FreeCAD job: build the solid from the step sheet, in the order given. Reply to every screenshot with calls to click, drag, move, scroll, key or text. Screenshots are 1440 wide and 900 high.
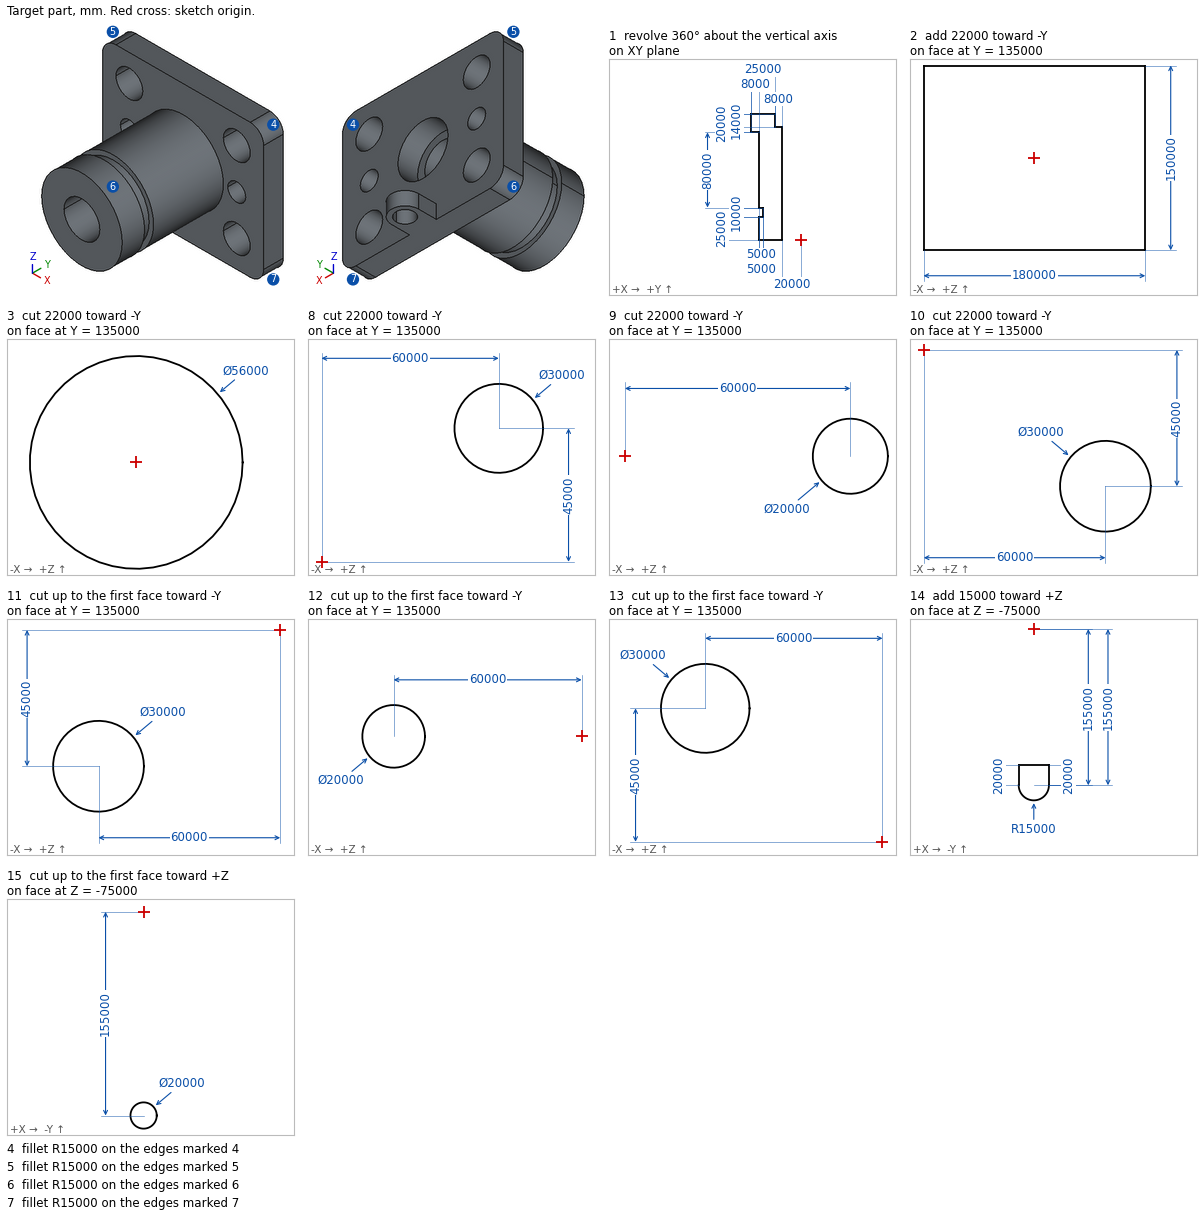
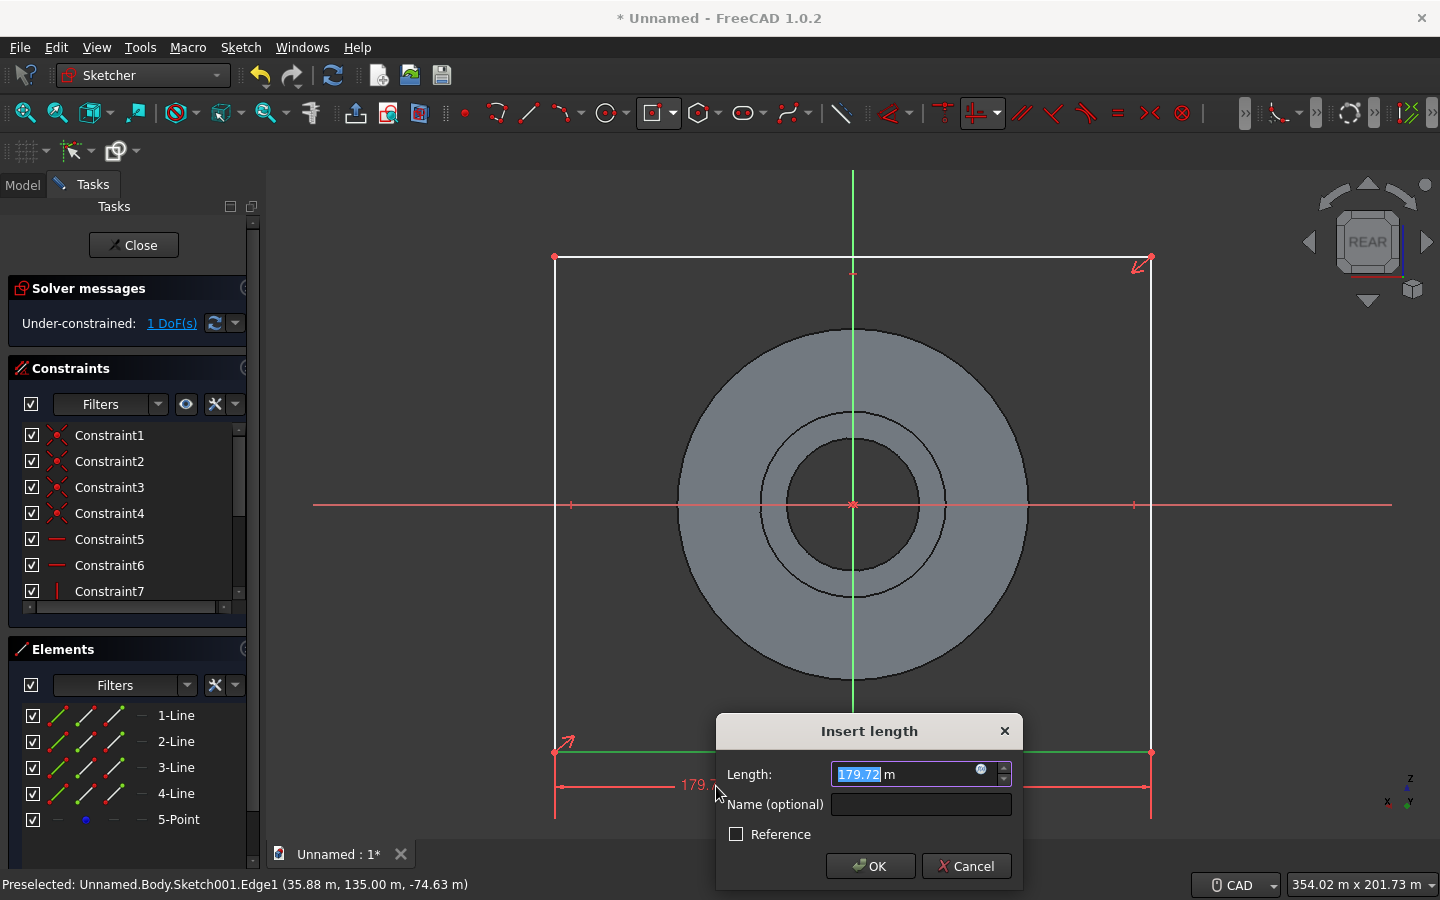
key(ctrl+a)
text(180000 mm)
key(Return)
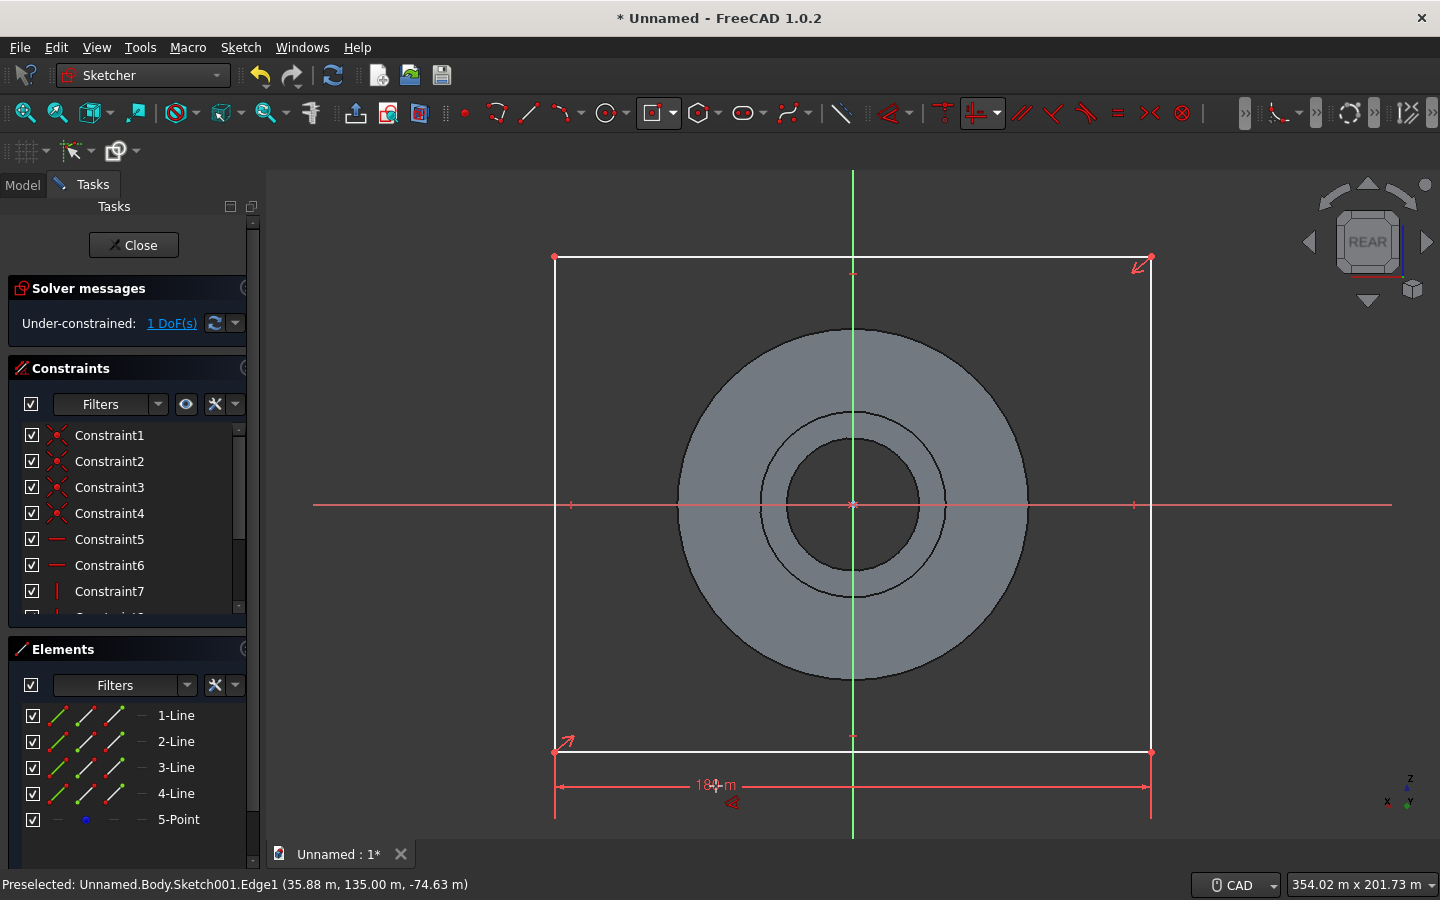
click(1151, 604)
click(1185, 391)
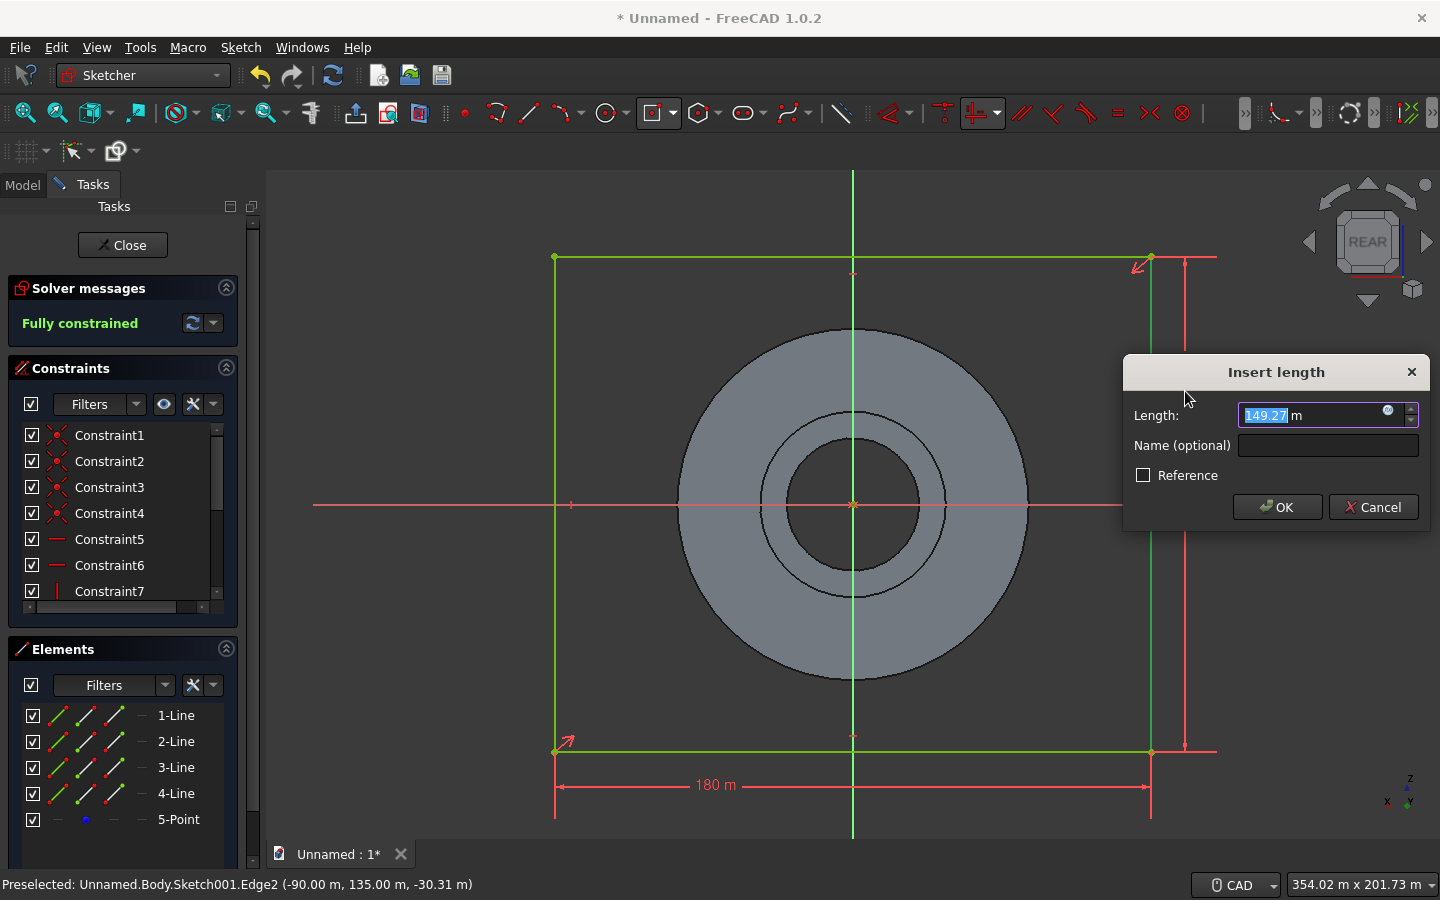
key(ctrl+a)
text(150000 mm)
key(Return)
key(Escape)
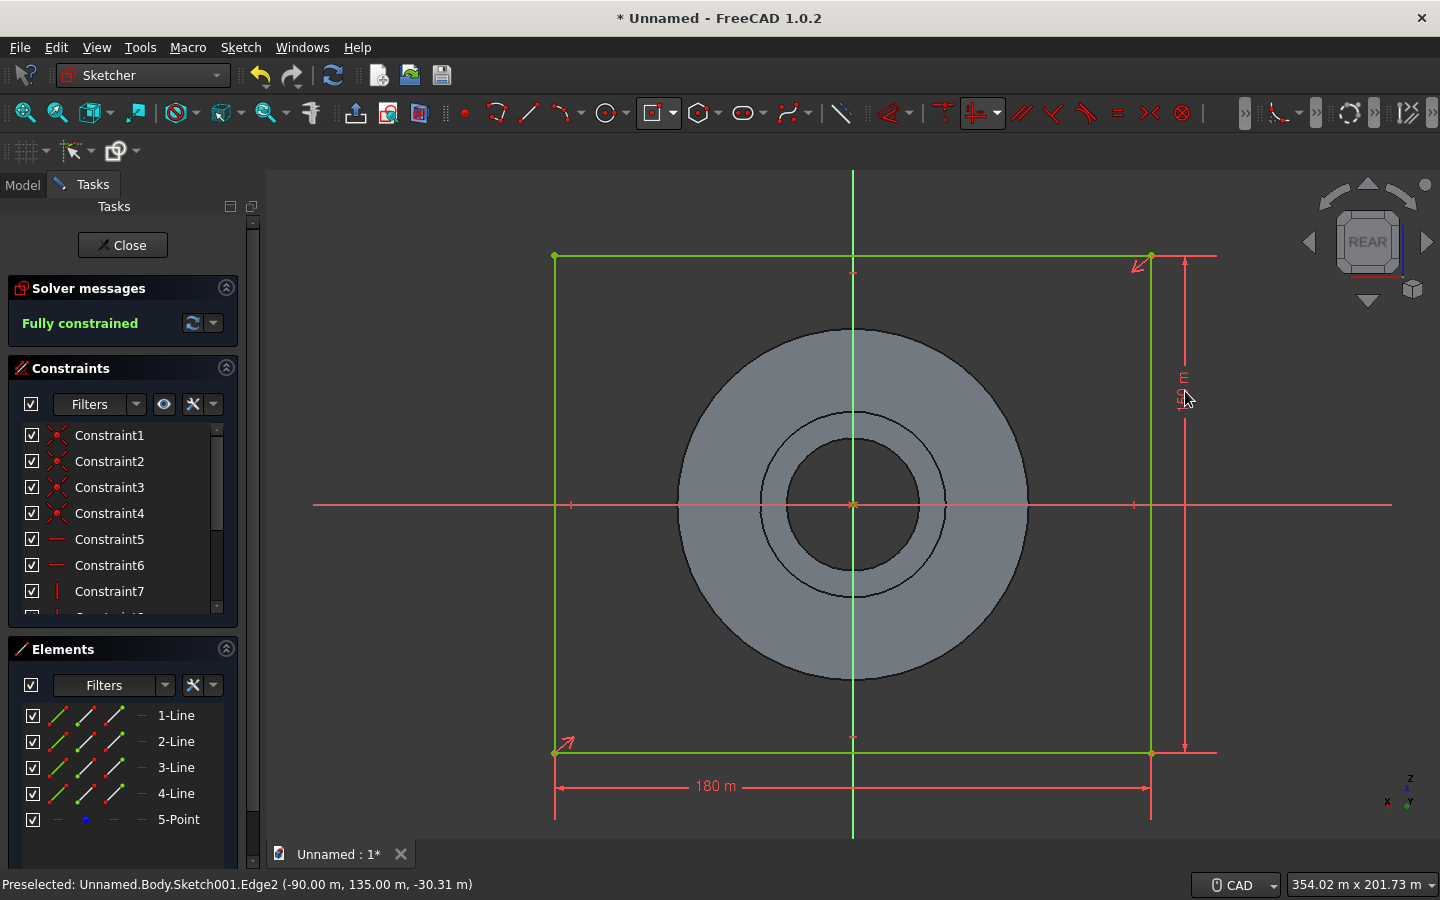
click(123, 245)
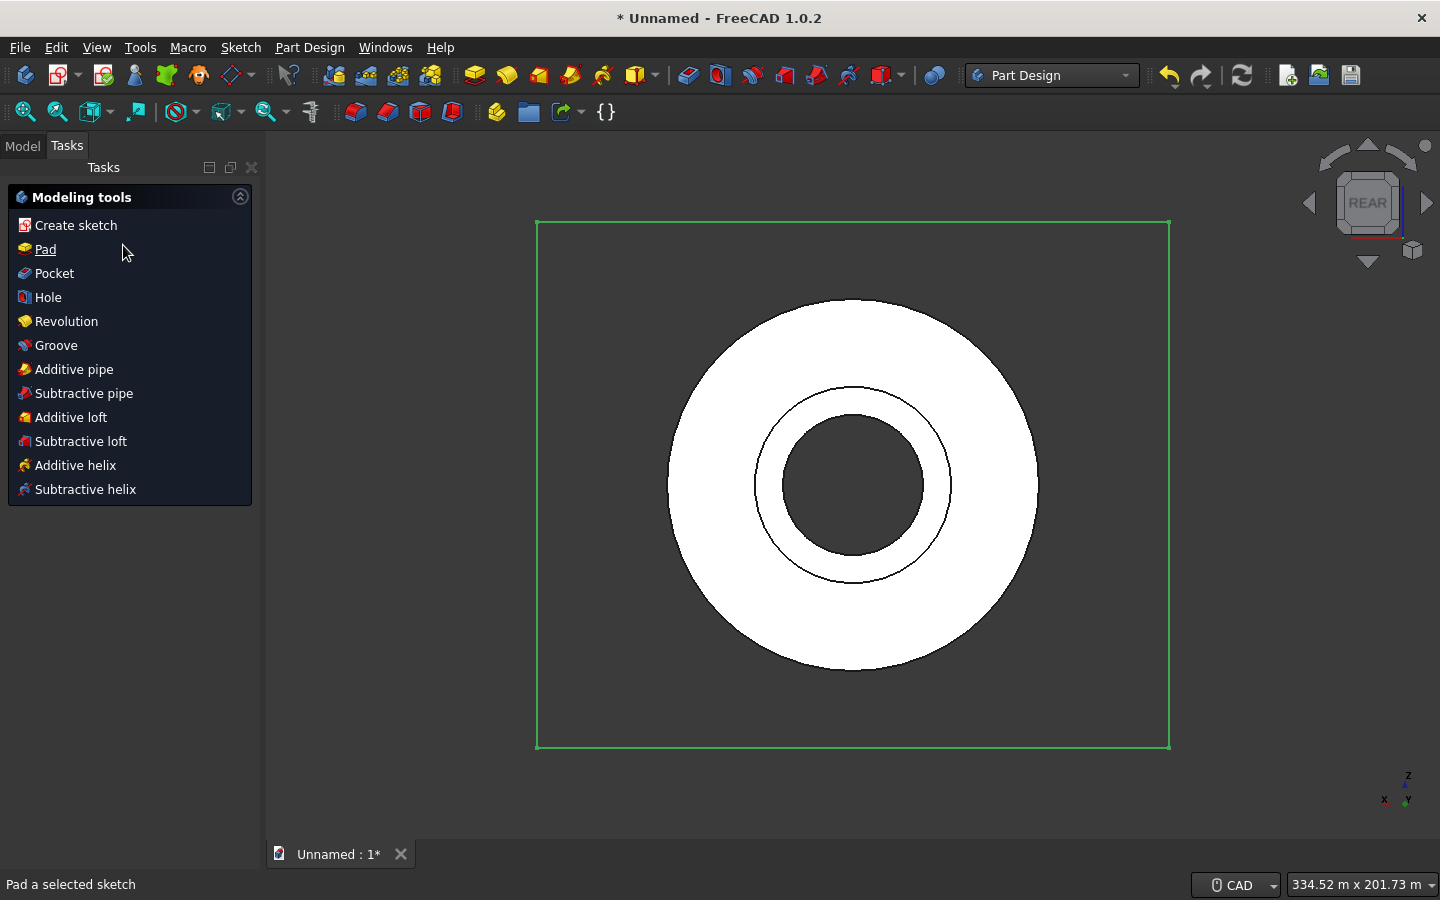
click(476, 76)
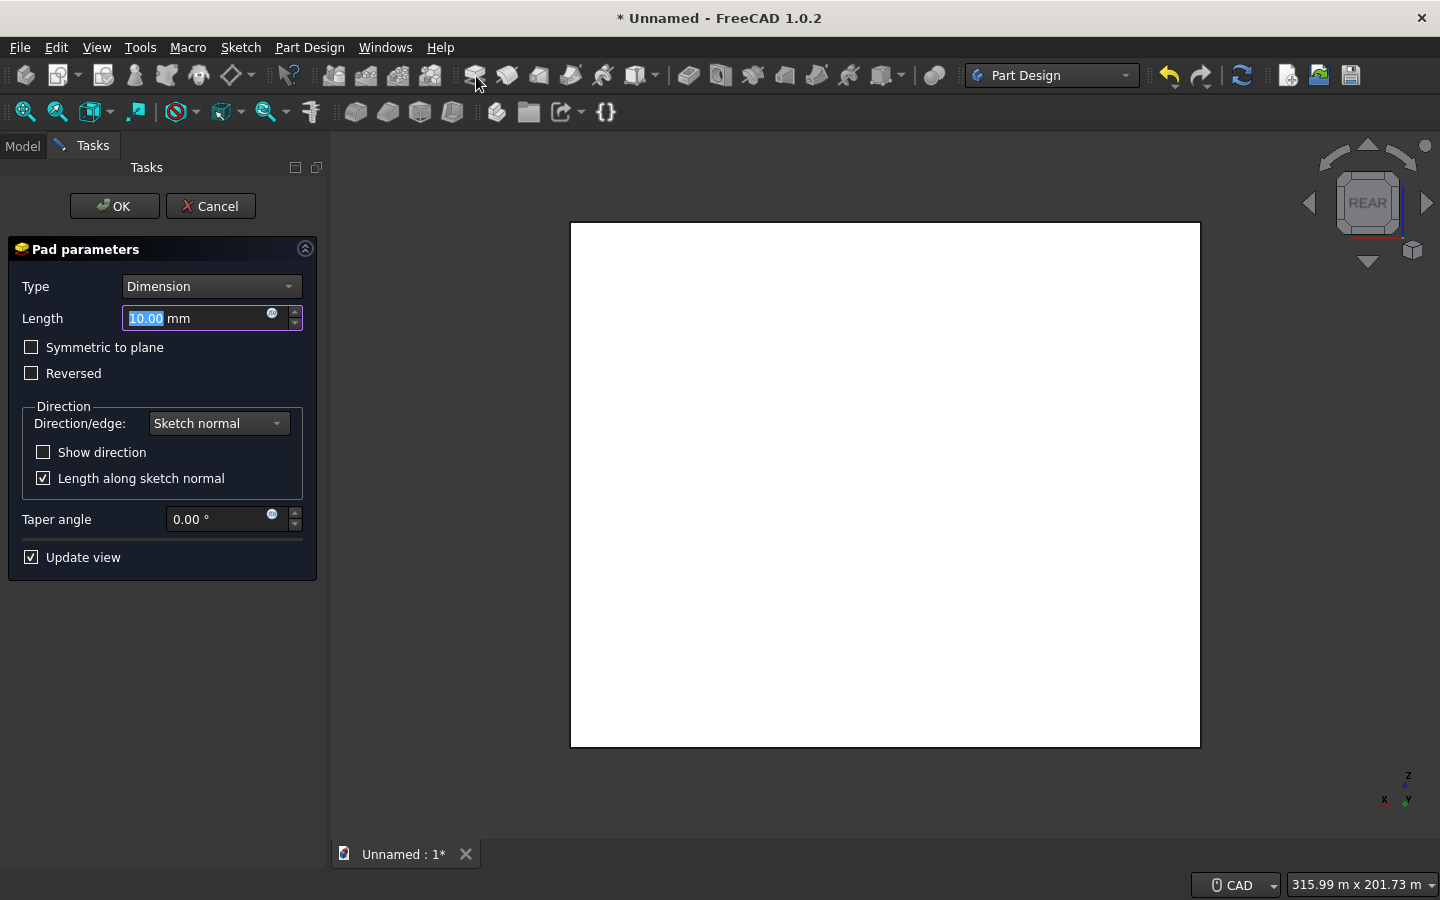
text(22000)
key(Tab)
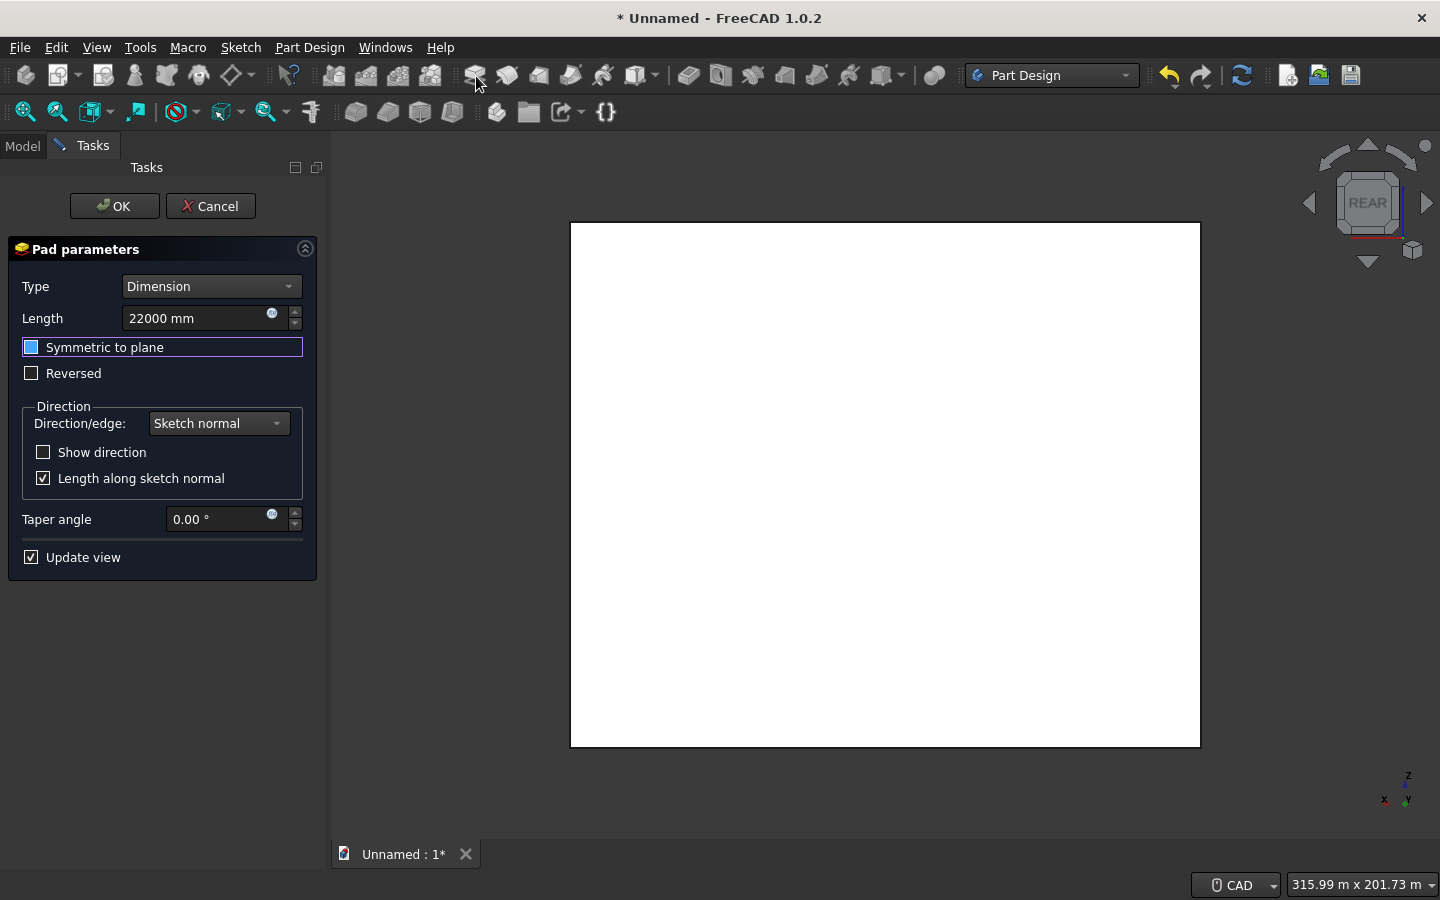
click(30, 373)